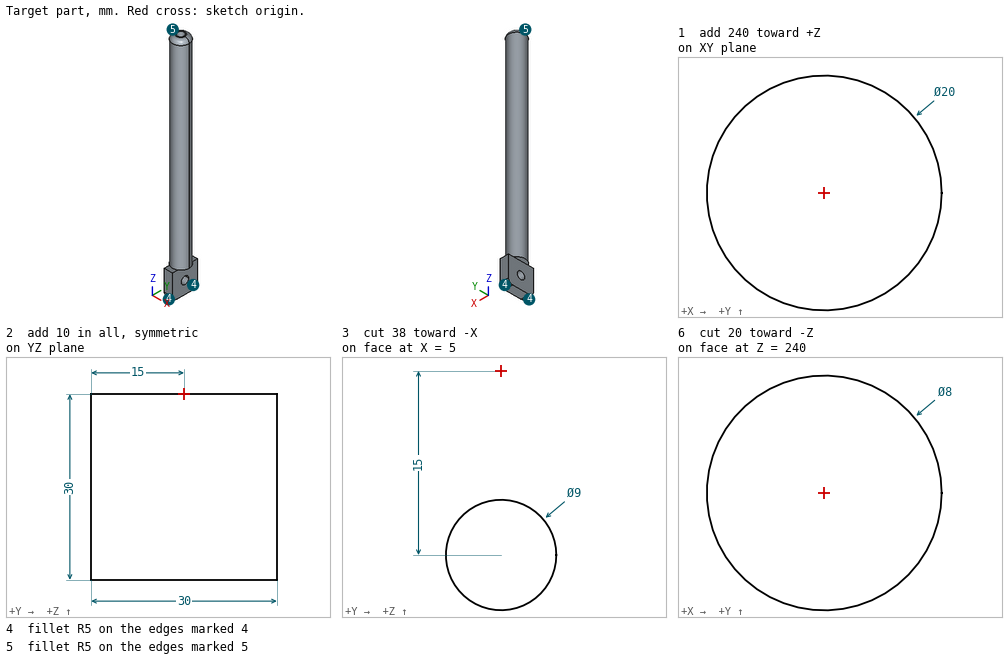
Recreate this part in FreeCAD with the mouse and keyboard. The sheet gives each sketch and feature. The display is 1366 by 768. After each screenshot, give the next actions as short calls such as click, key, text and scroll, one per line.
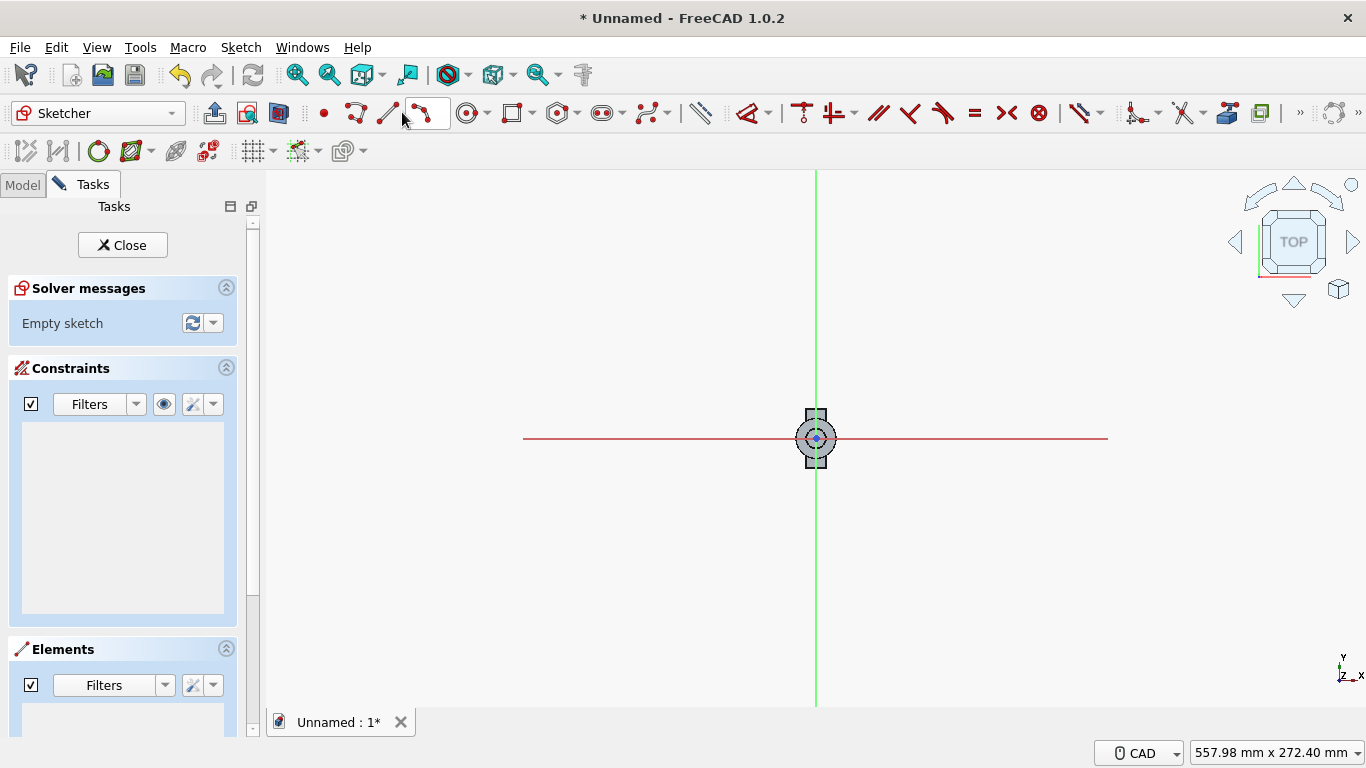
scroll(820, 438, up, 15)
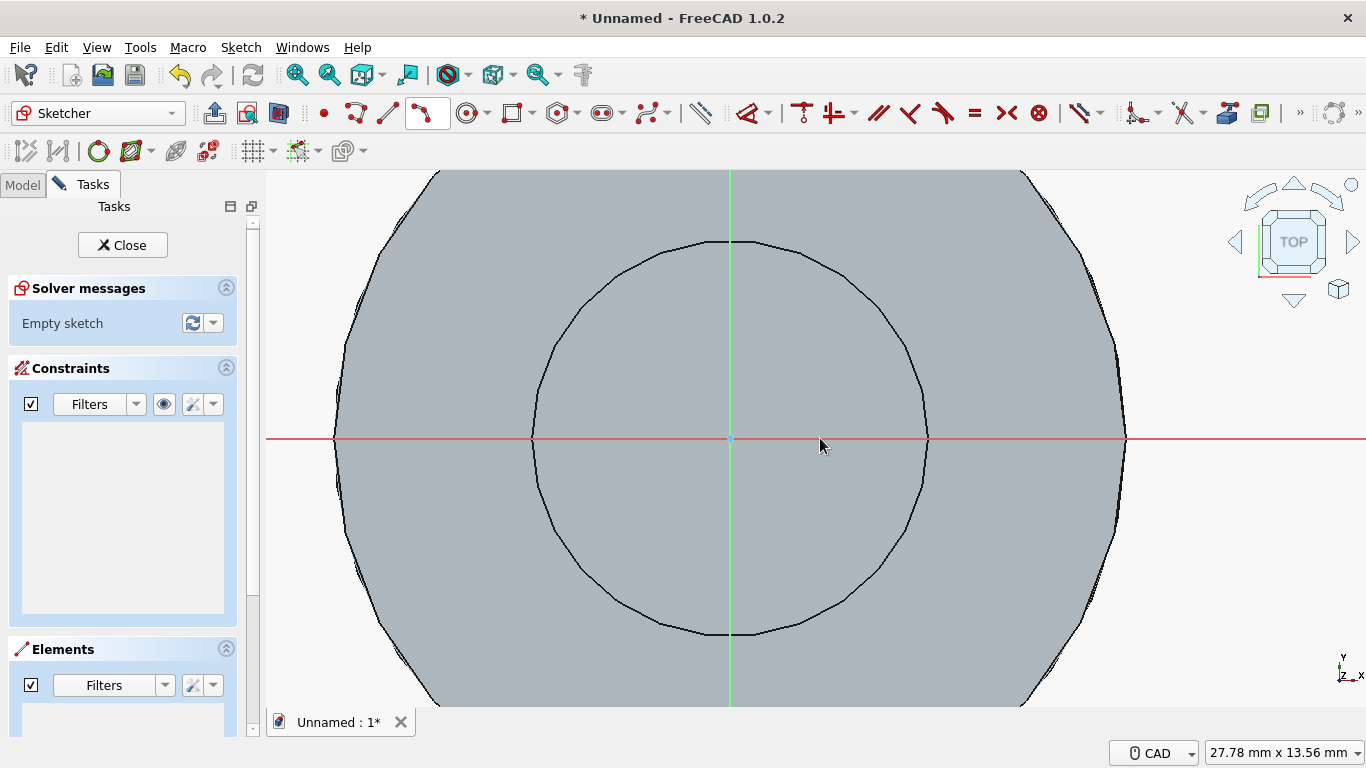
click(468, 114)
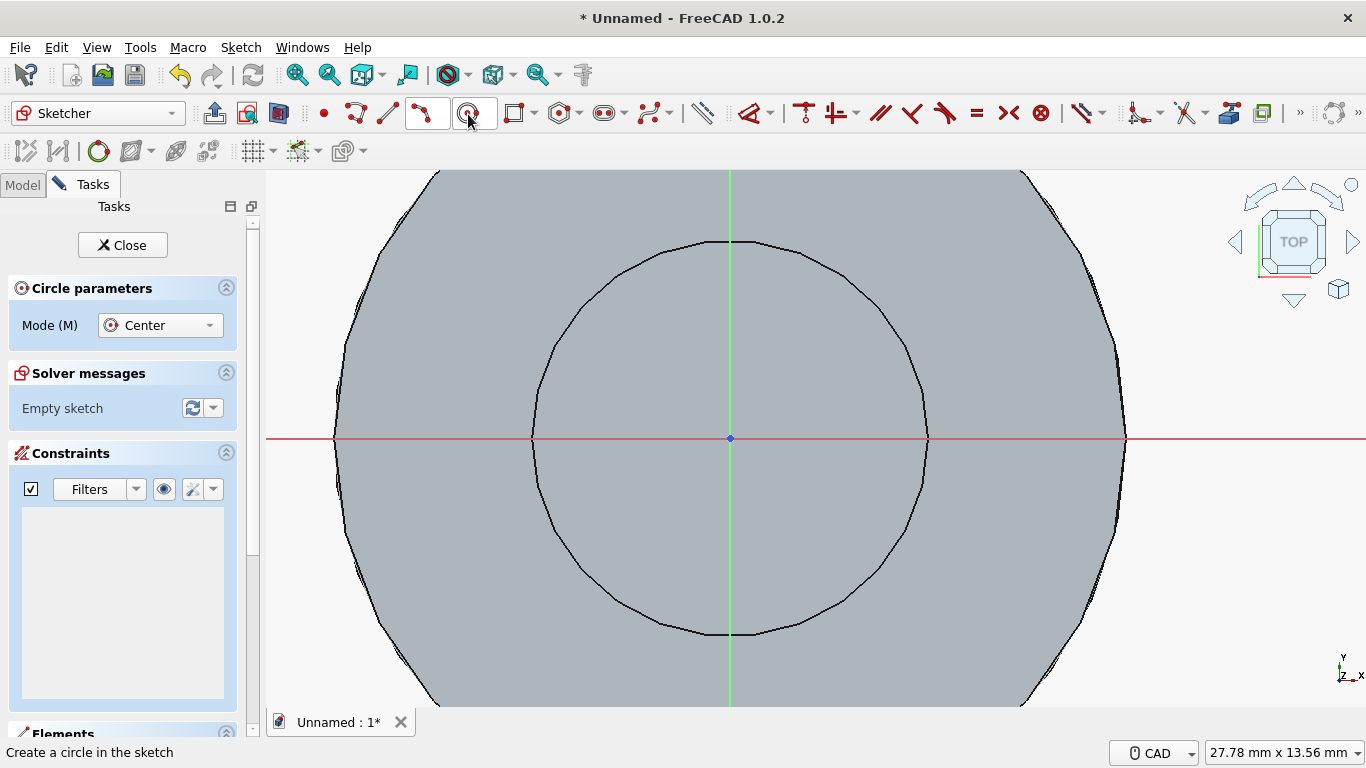
click(730, 438)
click(842, 327)
key(Escape)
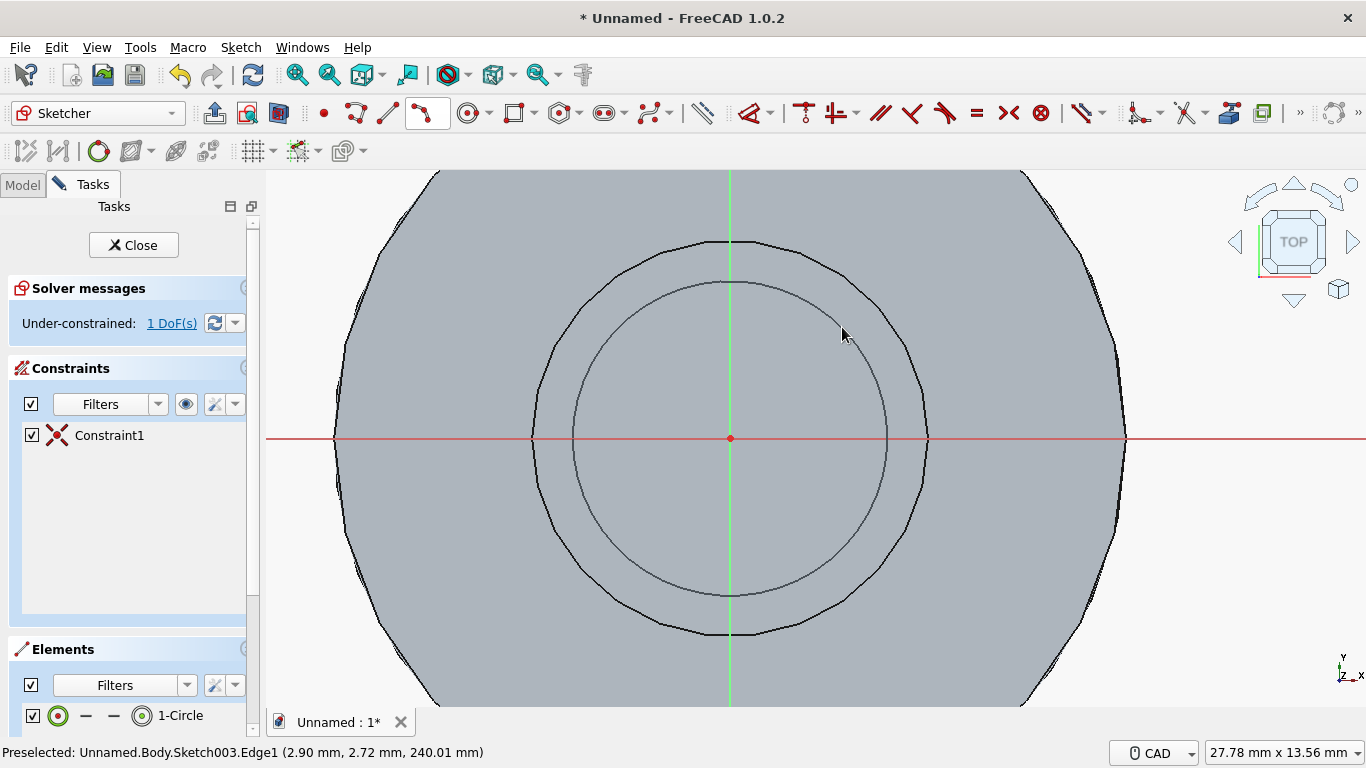
key(d)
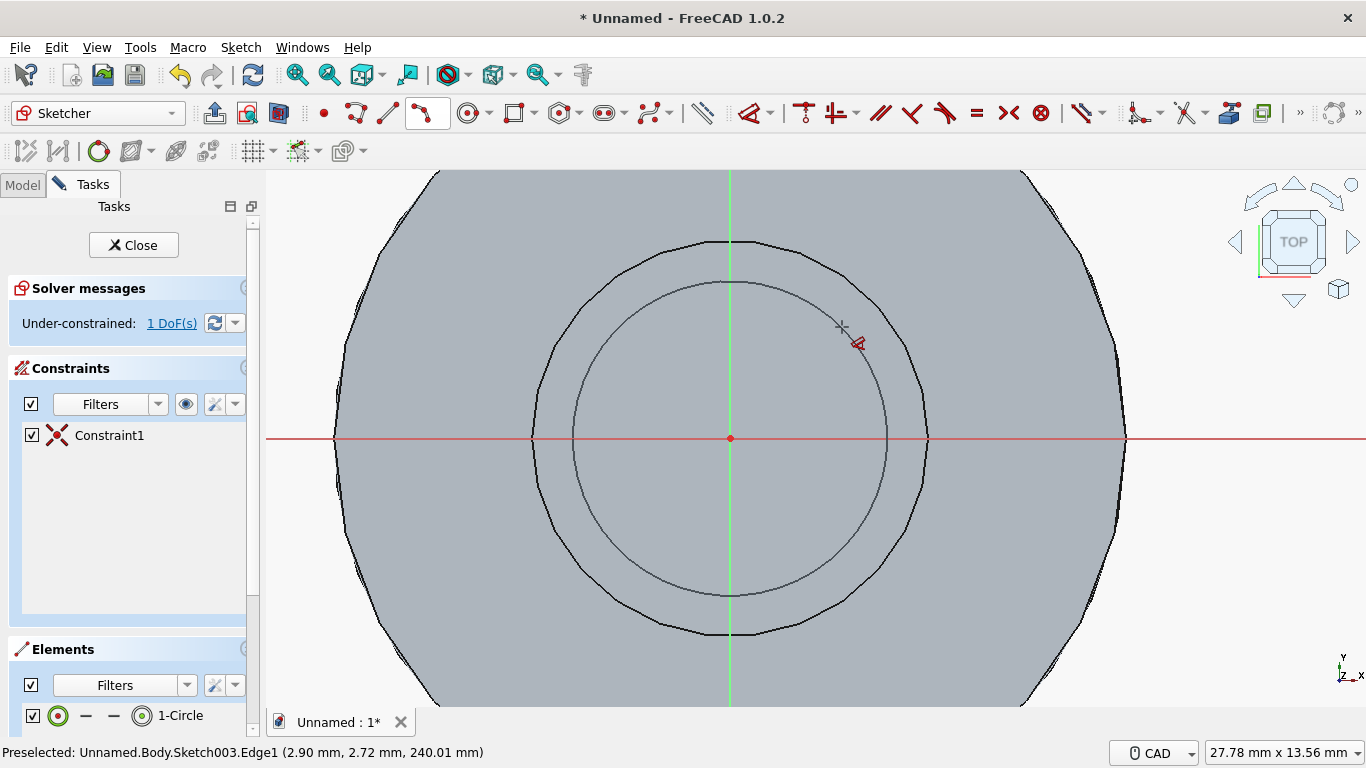
click(841, 327)
click(864, 304)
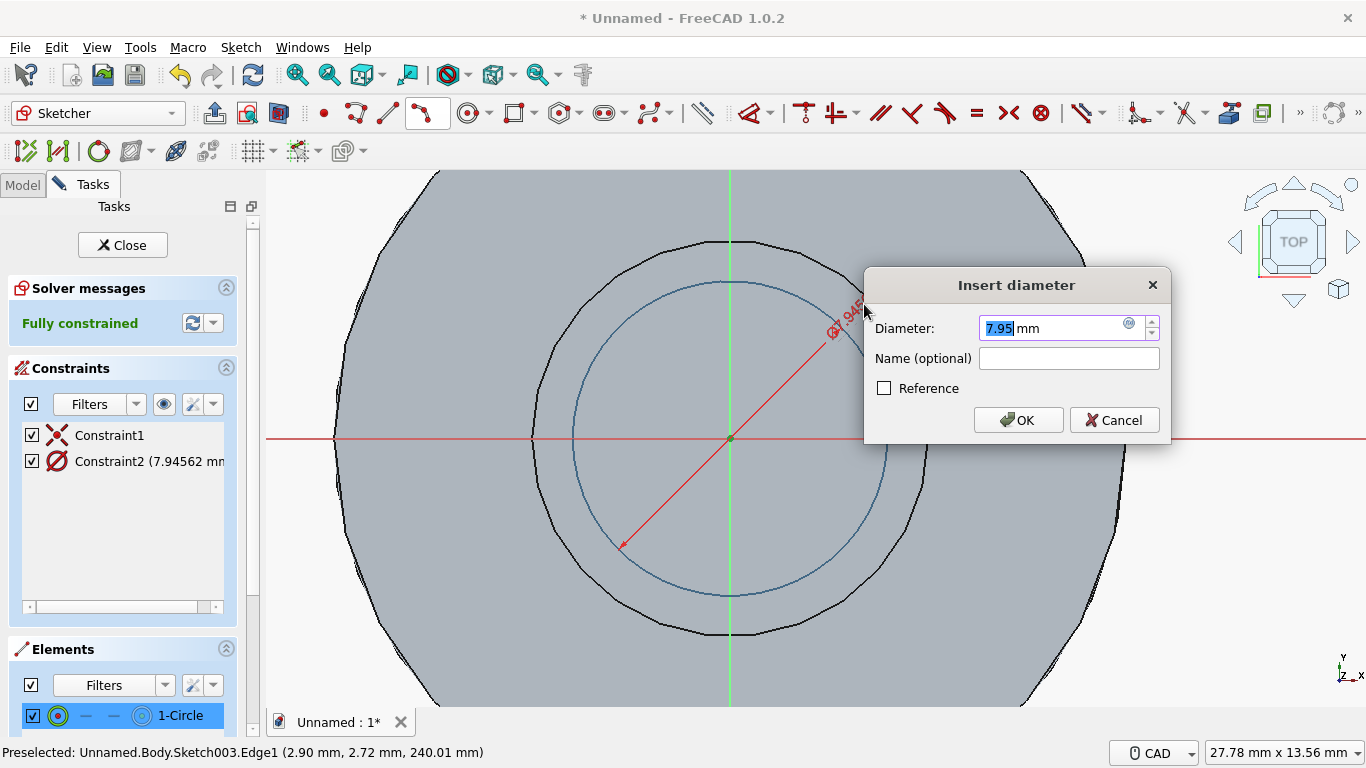
text(8)
key(Return)
key(Escape)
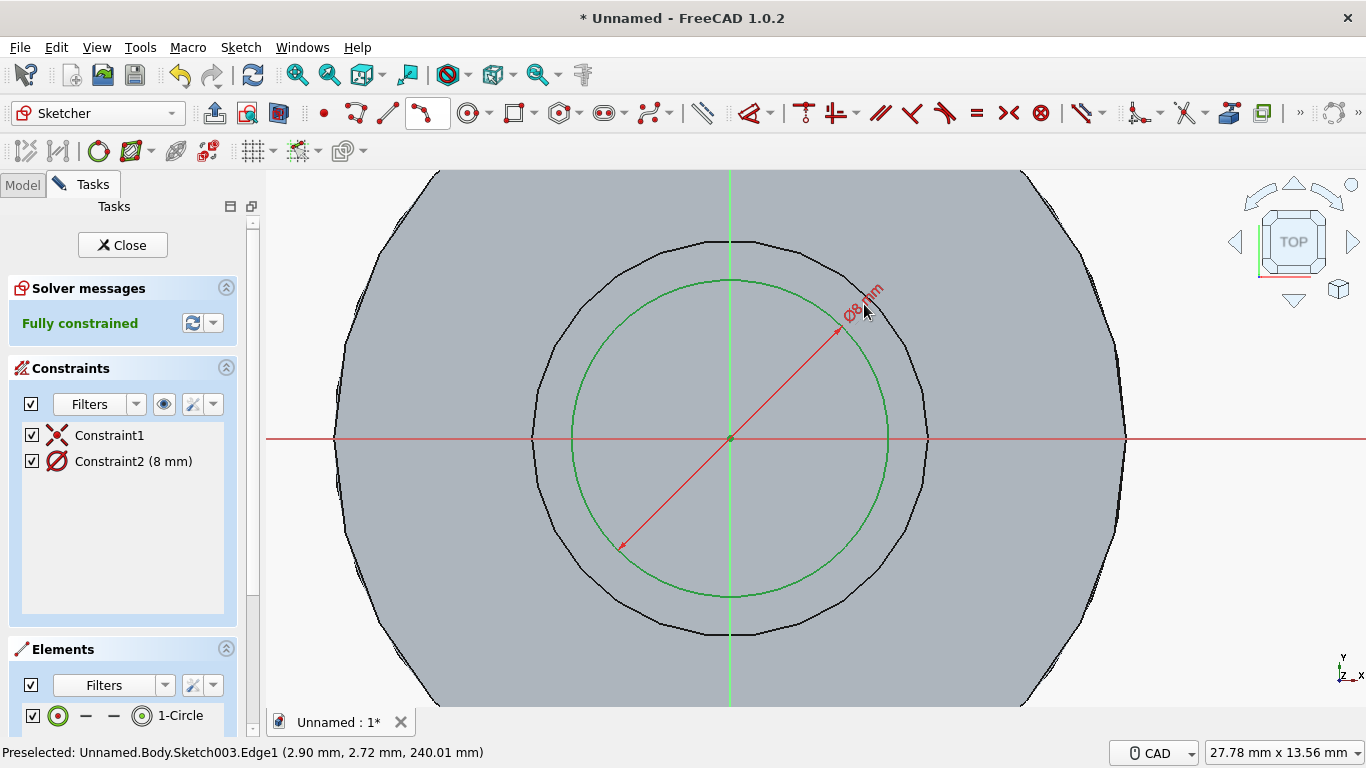
click(123, 245)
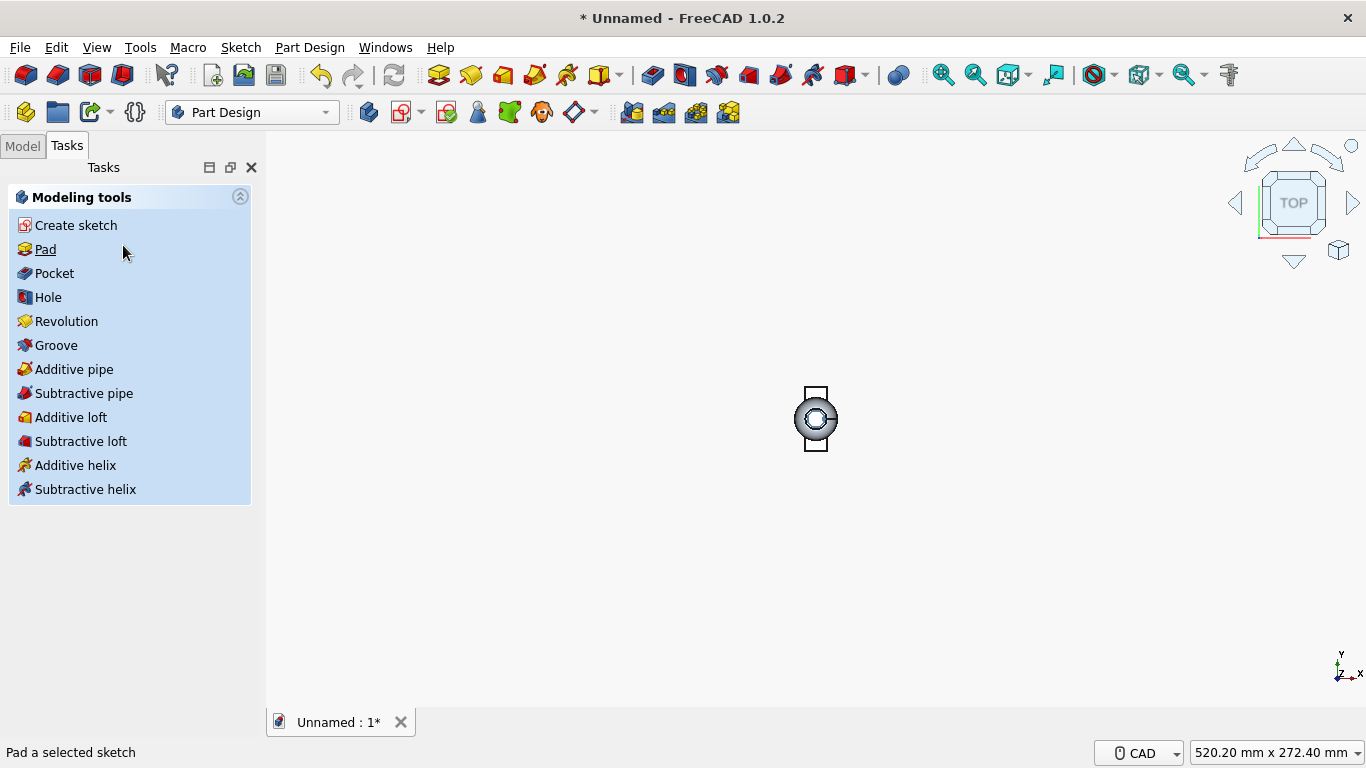
click(654, 76)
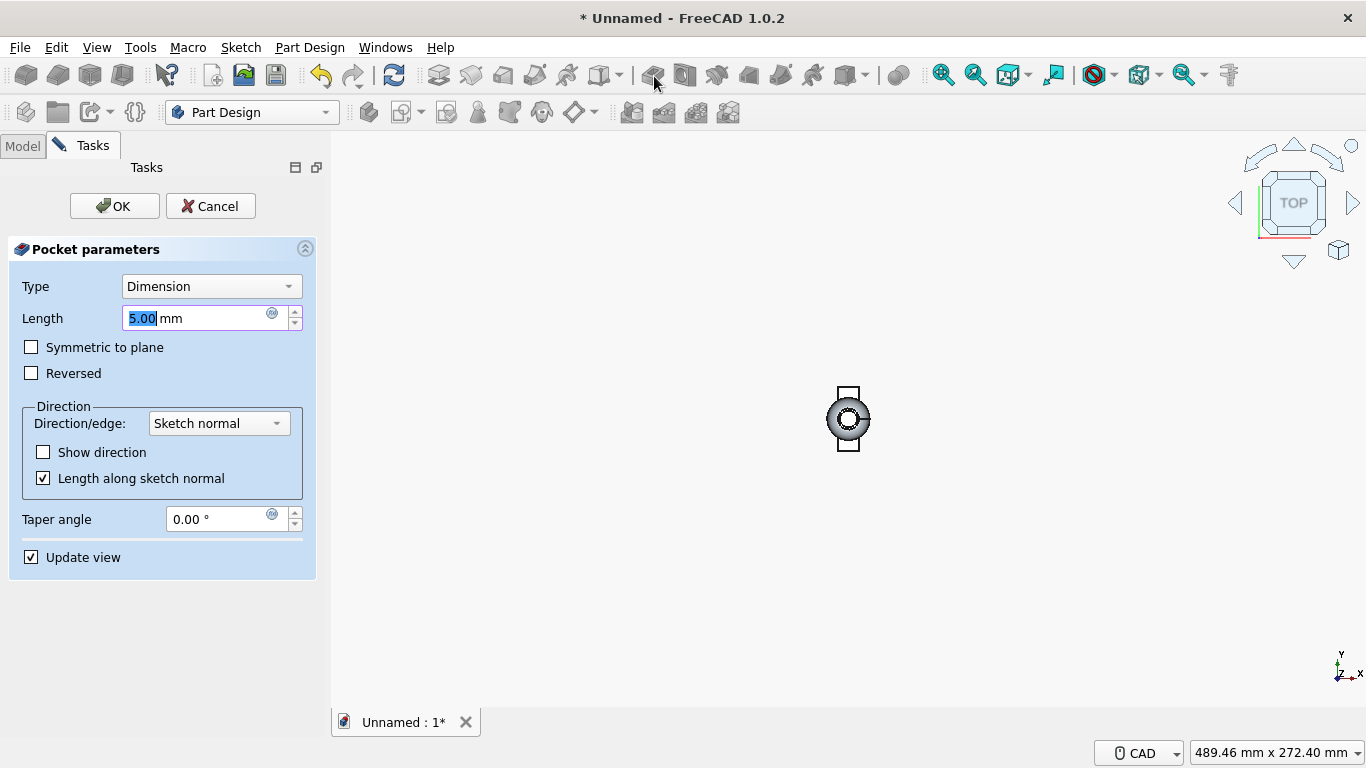
text(20)
key(Tab)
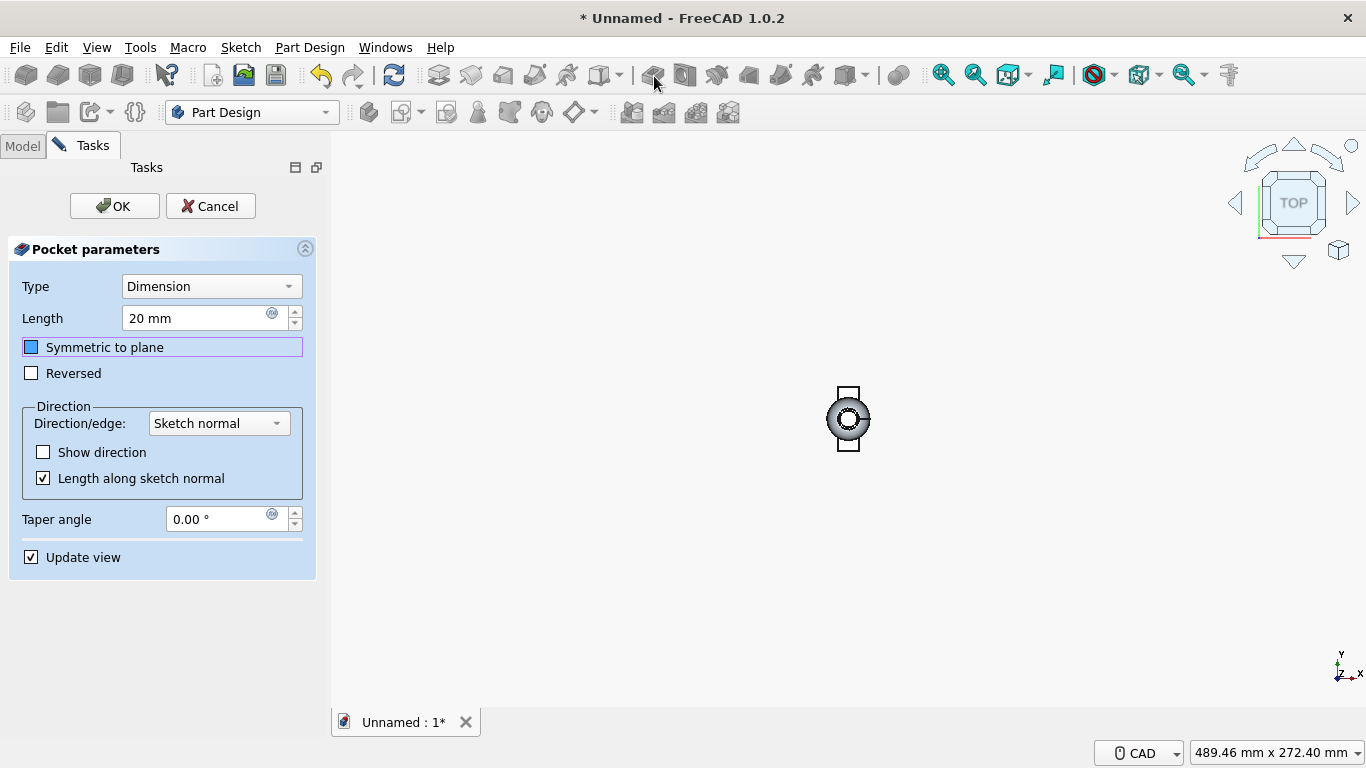
click(115, 206)